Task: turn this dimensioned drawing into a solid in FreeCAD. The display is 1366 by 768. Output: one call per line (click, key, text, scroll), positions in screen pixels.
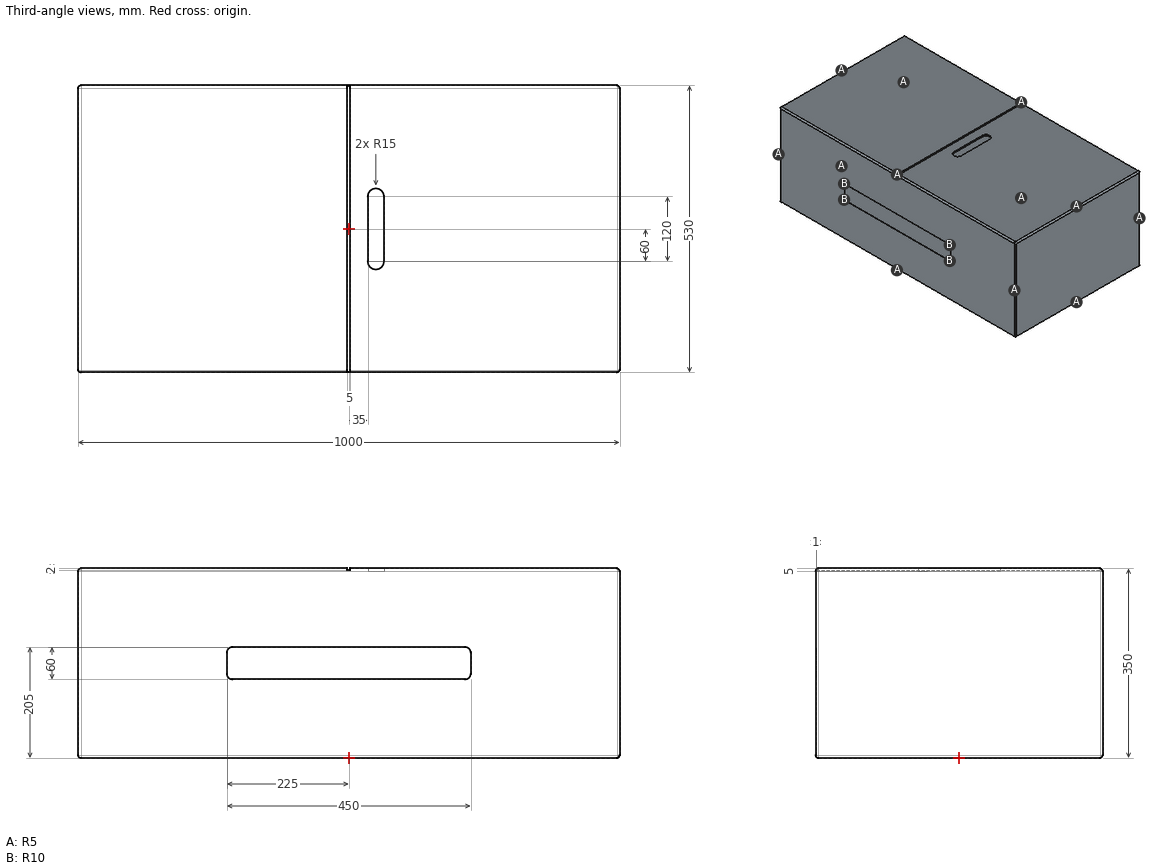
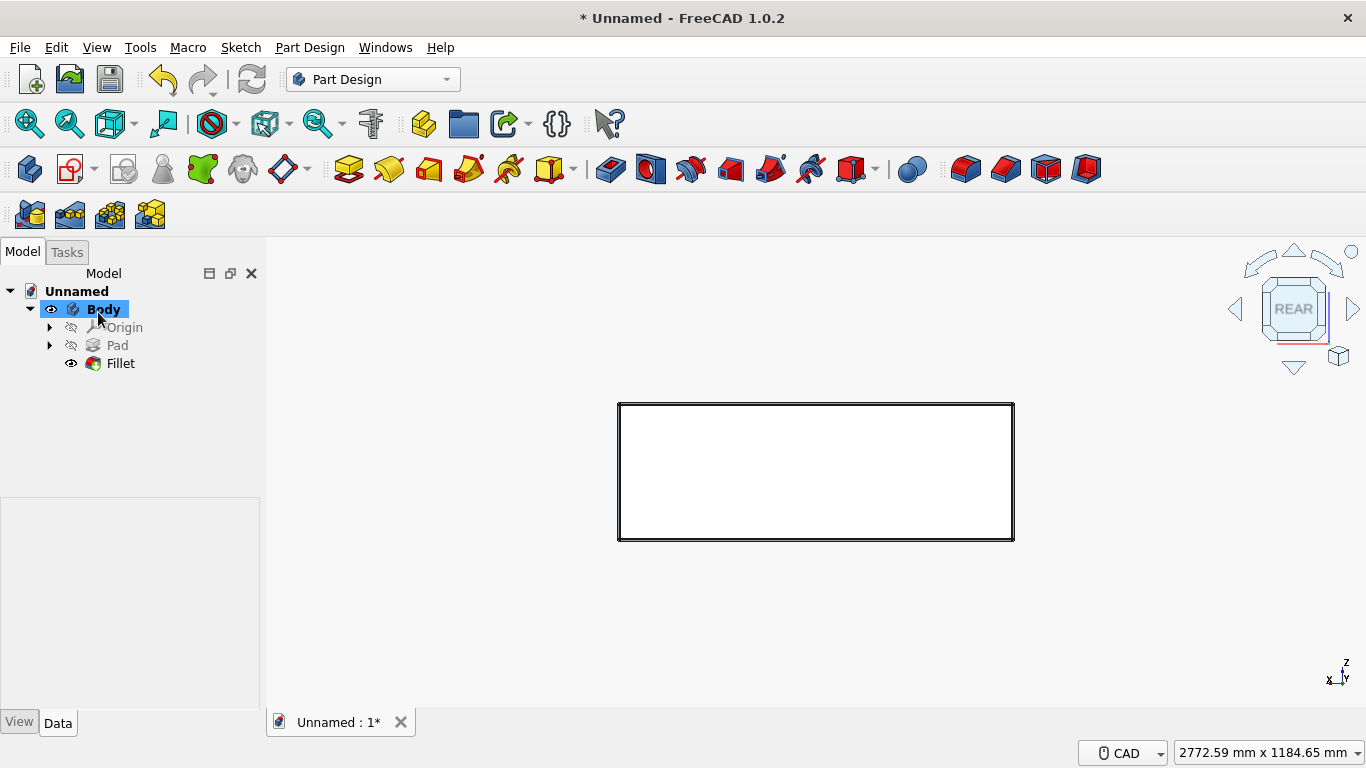
click(30, 124)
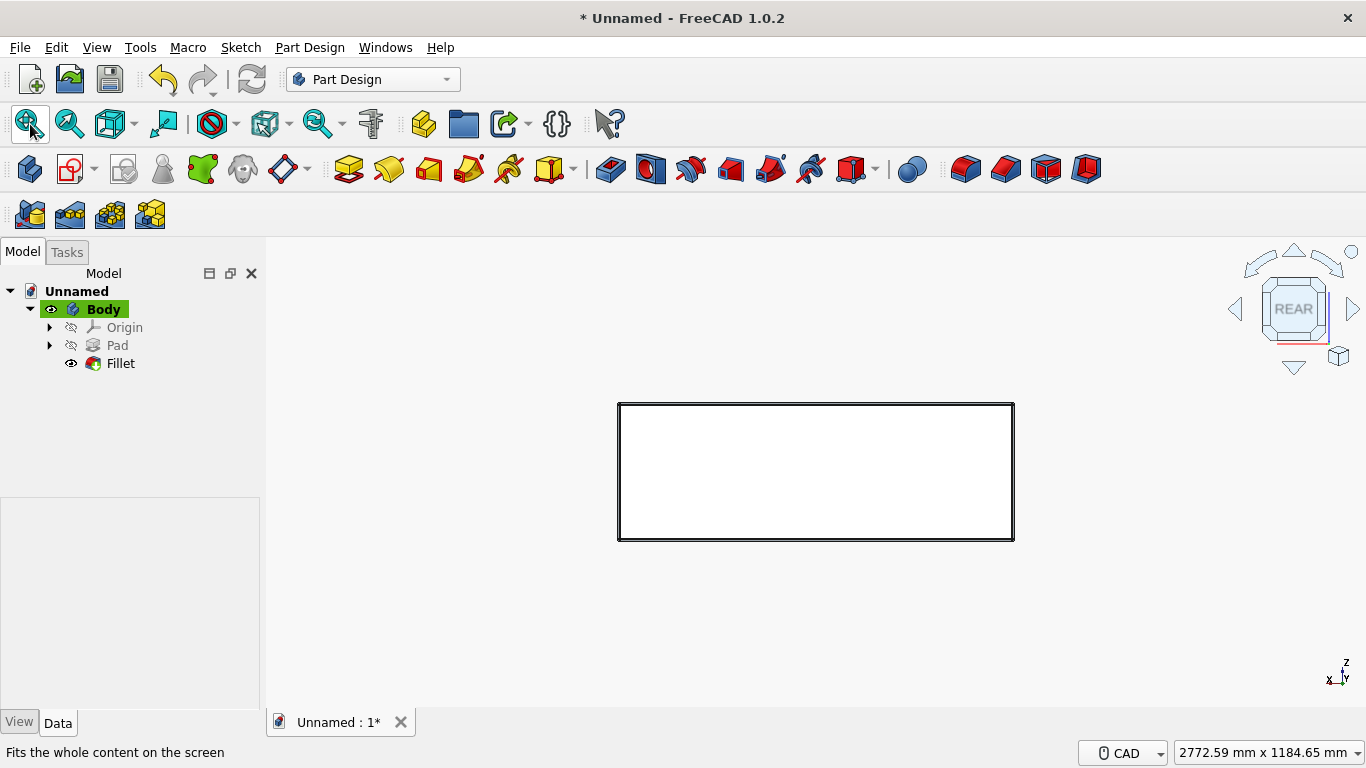
key(0)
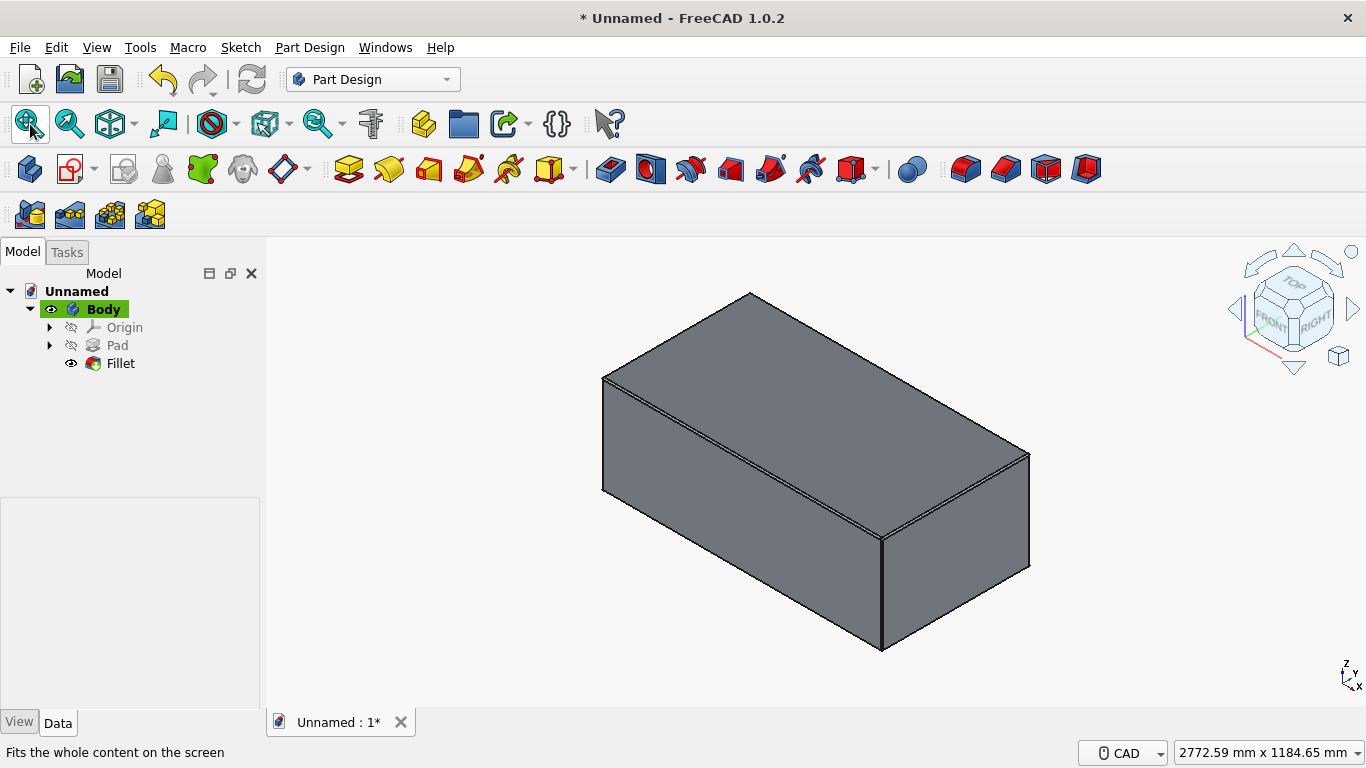
click(856, 437)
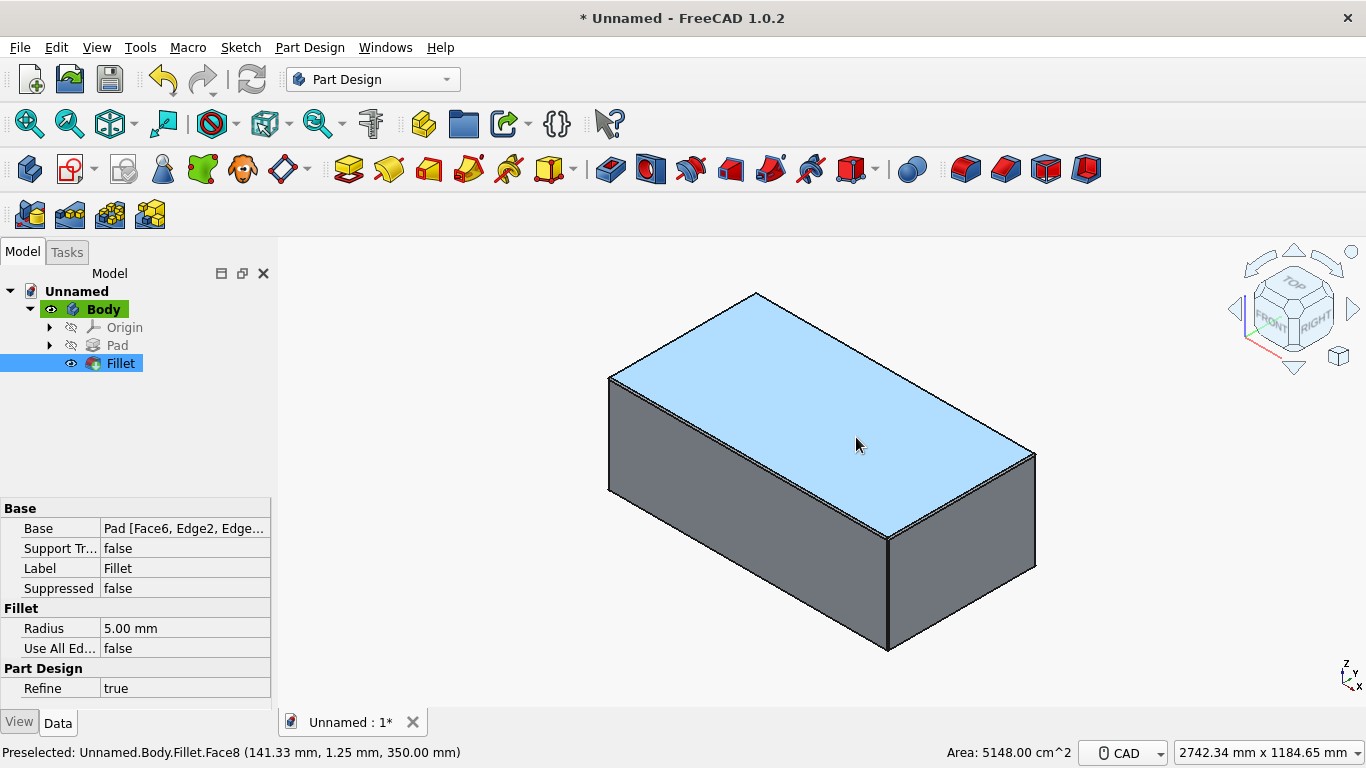
click(70, 170)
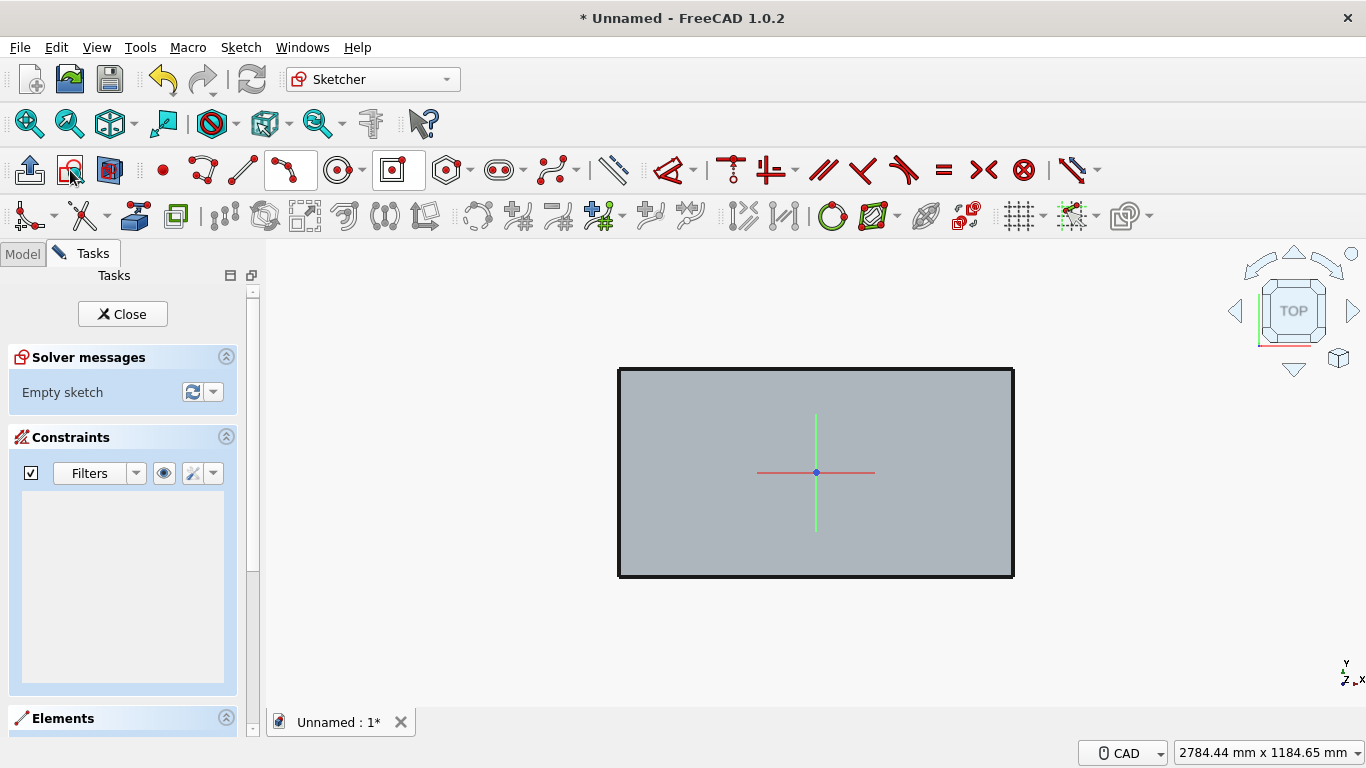
scroll(955, 473, up, 2)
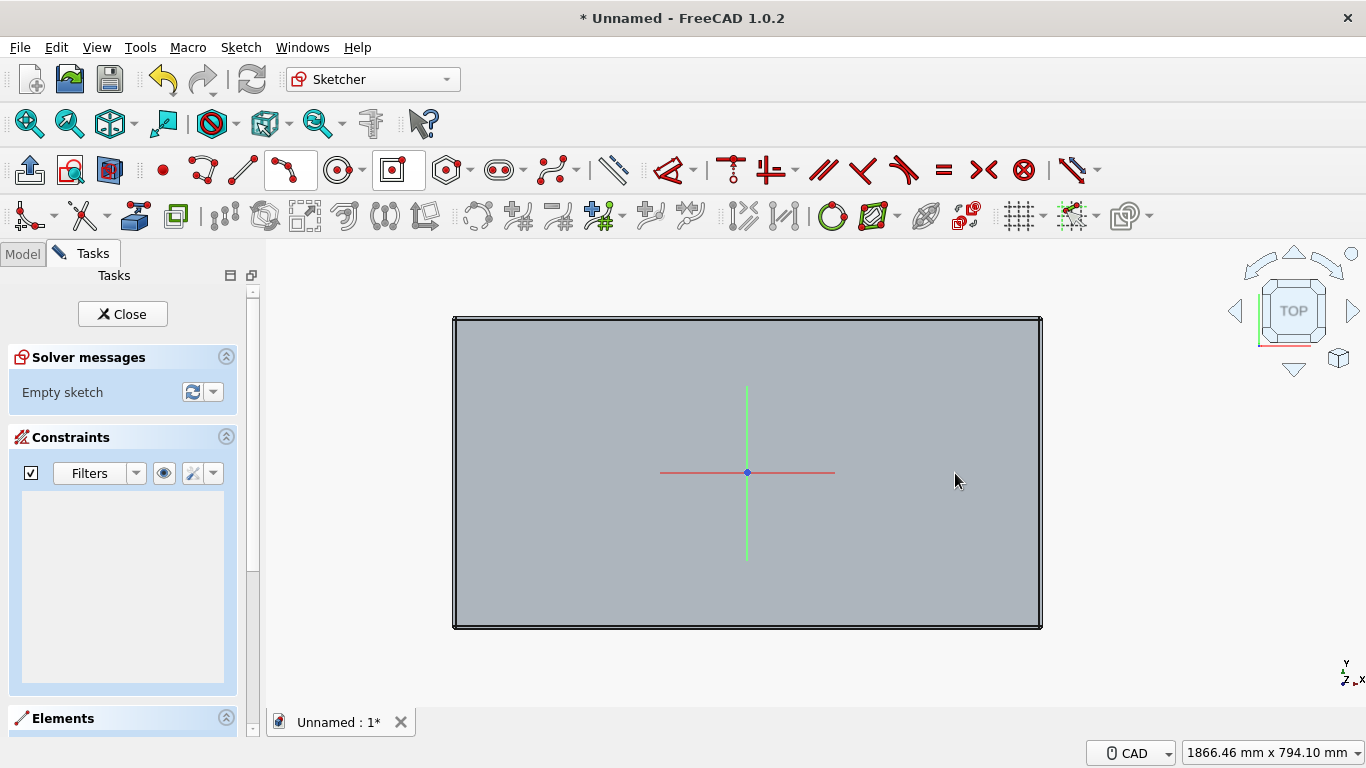
click(392, 170)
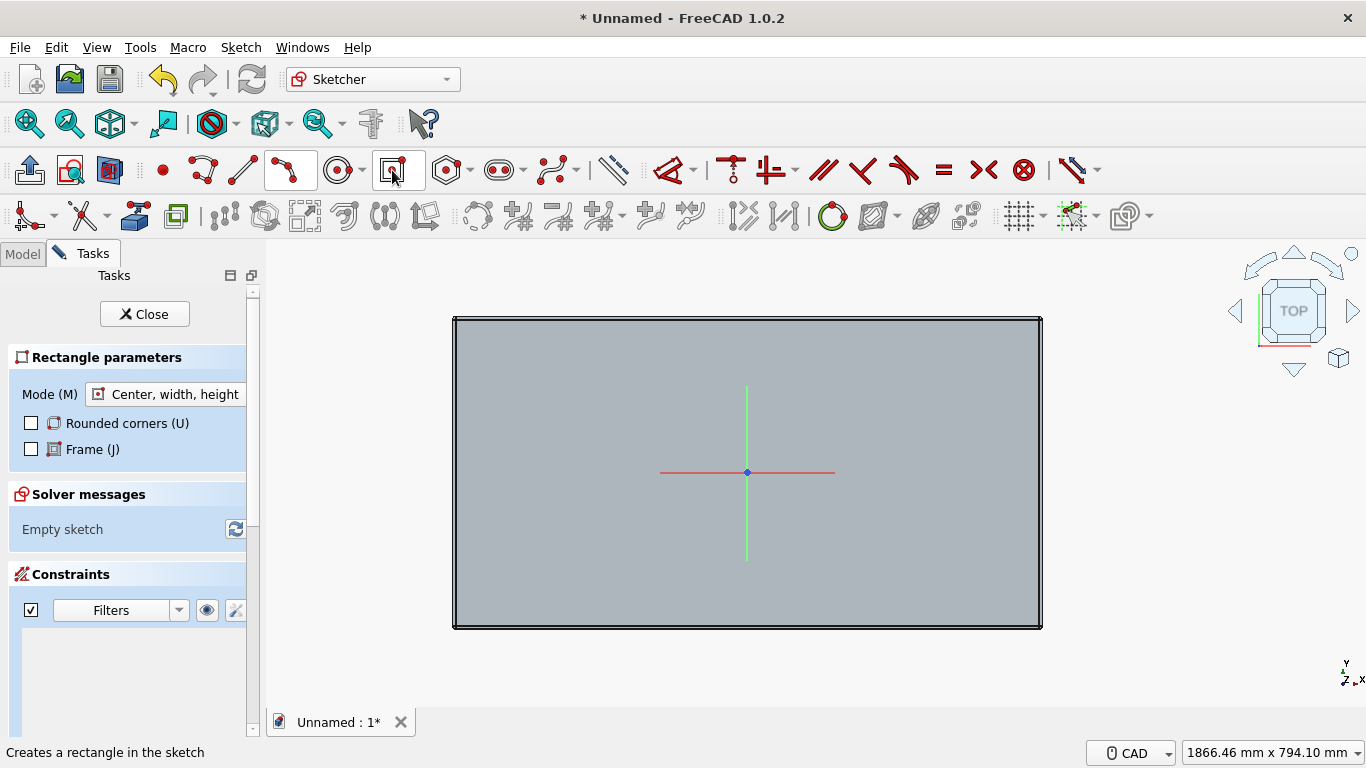
scroll(747, 473, up, 12)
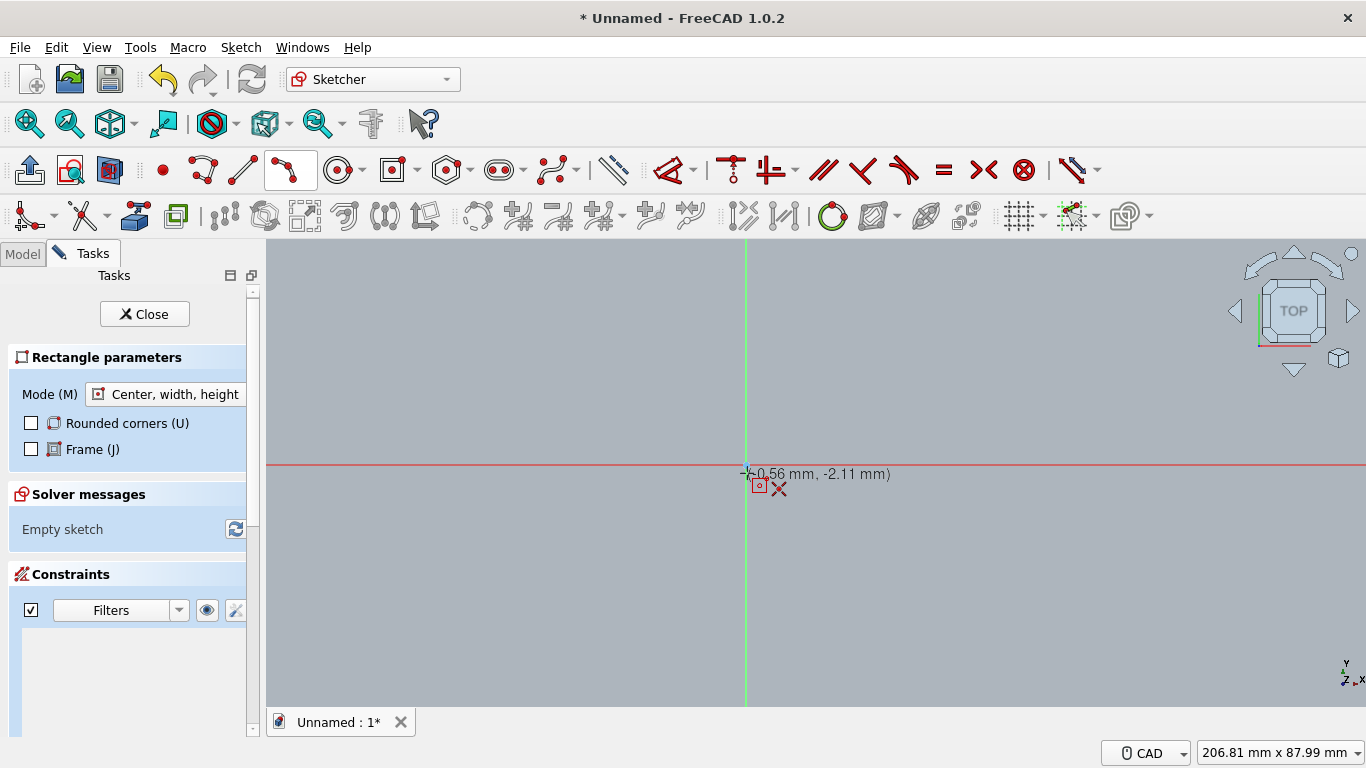
scroll(748, 474, down, 12)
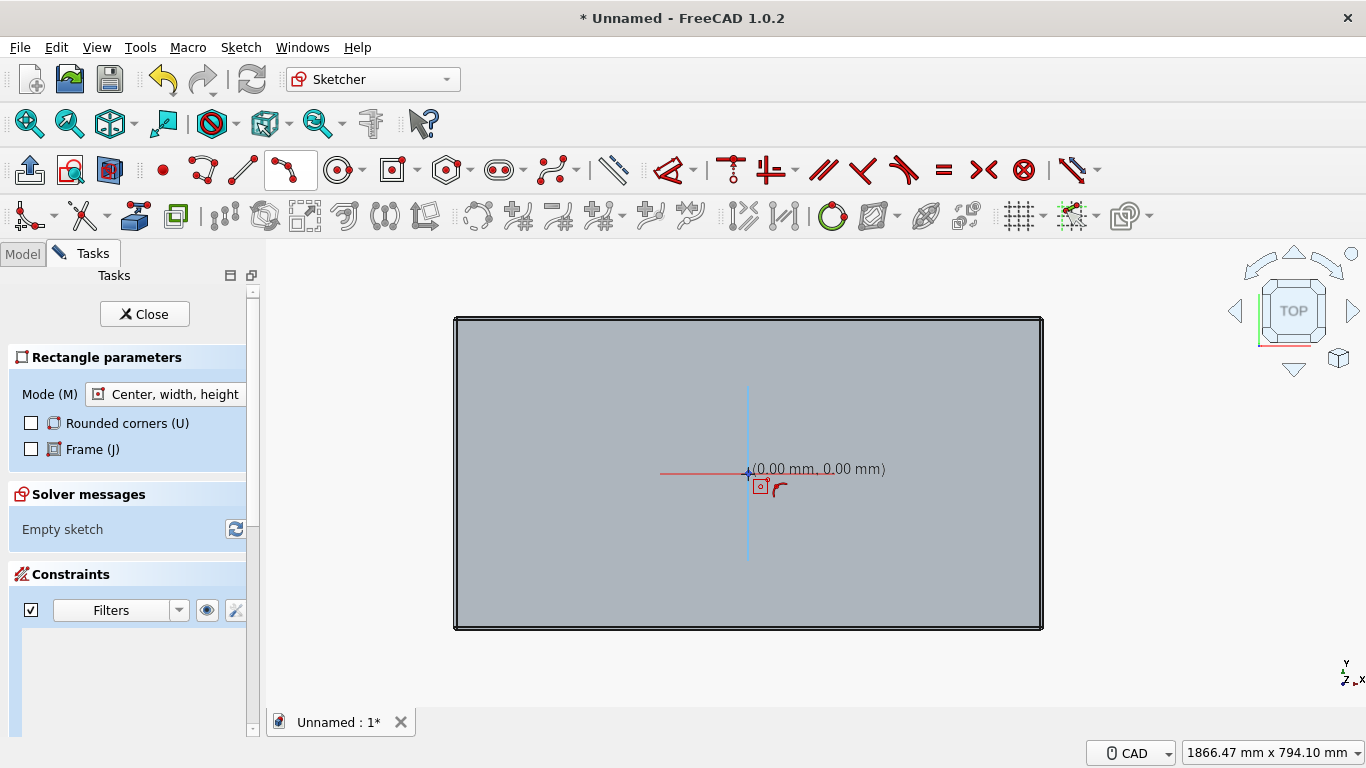
click(748, 474)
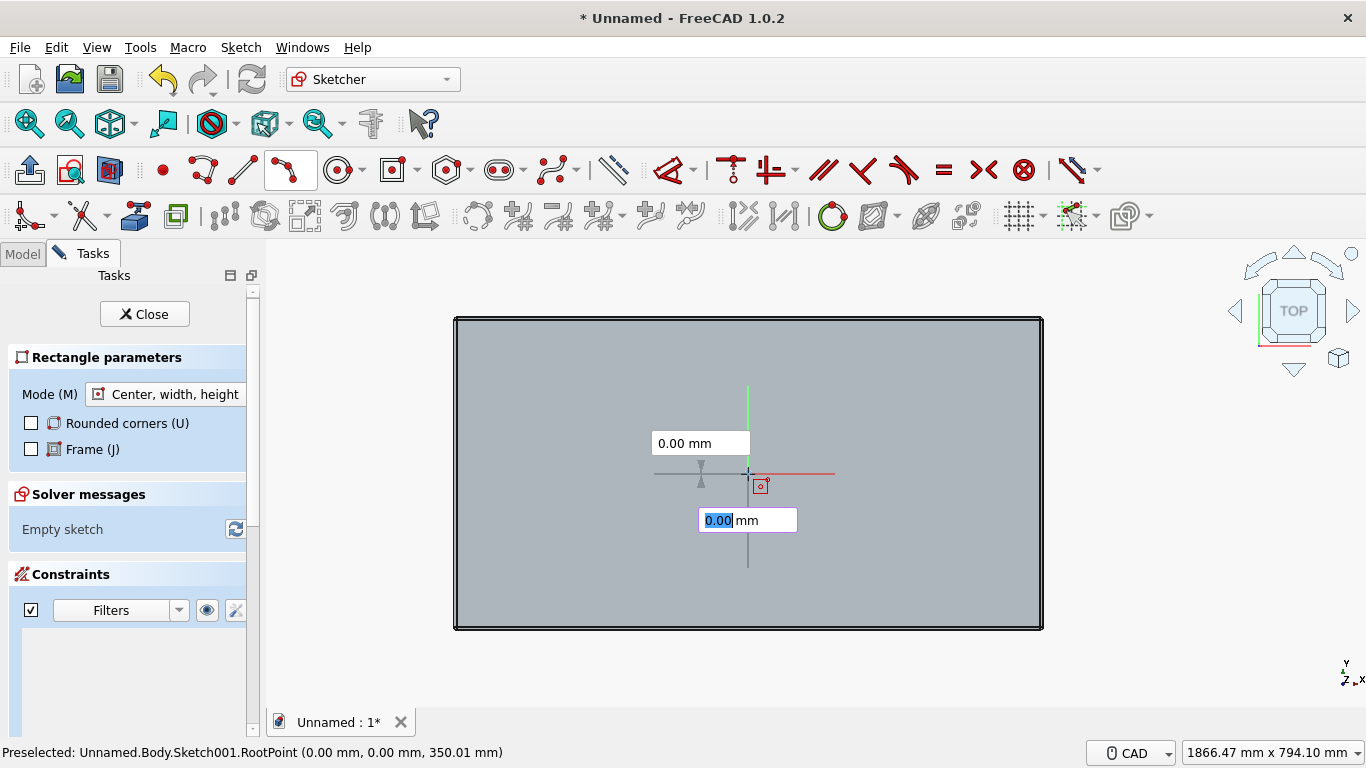
scroll(750, 317, up, 12)